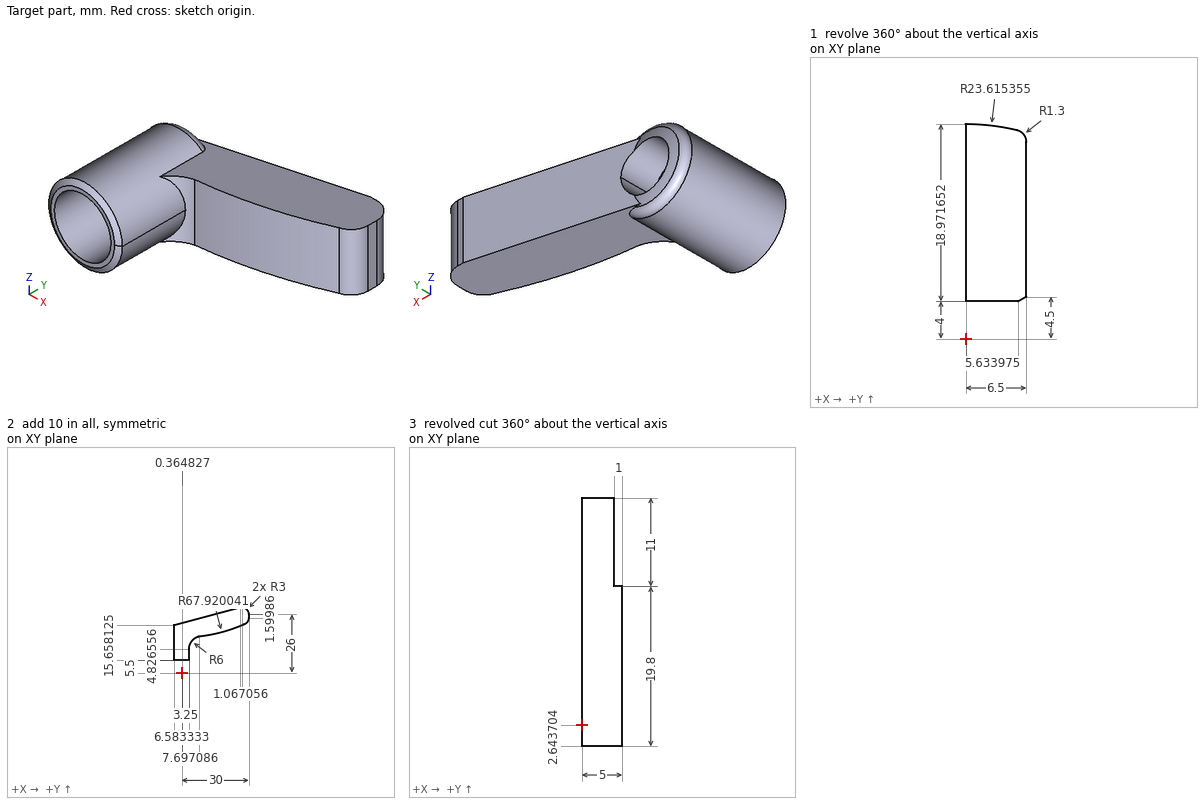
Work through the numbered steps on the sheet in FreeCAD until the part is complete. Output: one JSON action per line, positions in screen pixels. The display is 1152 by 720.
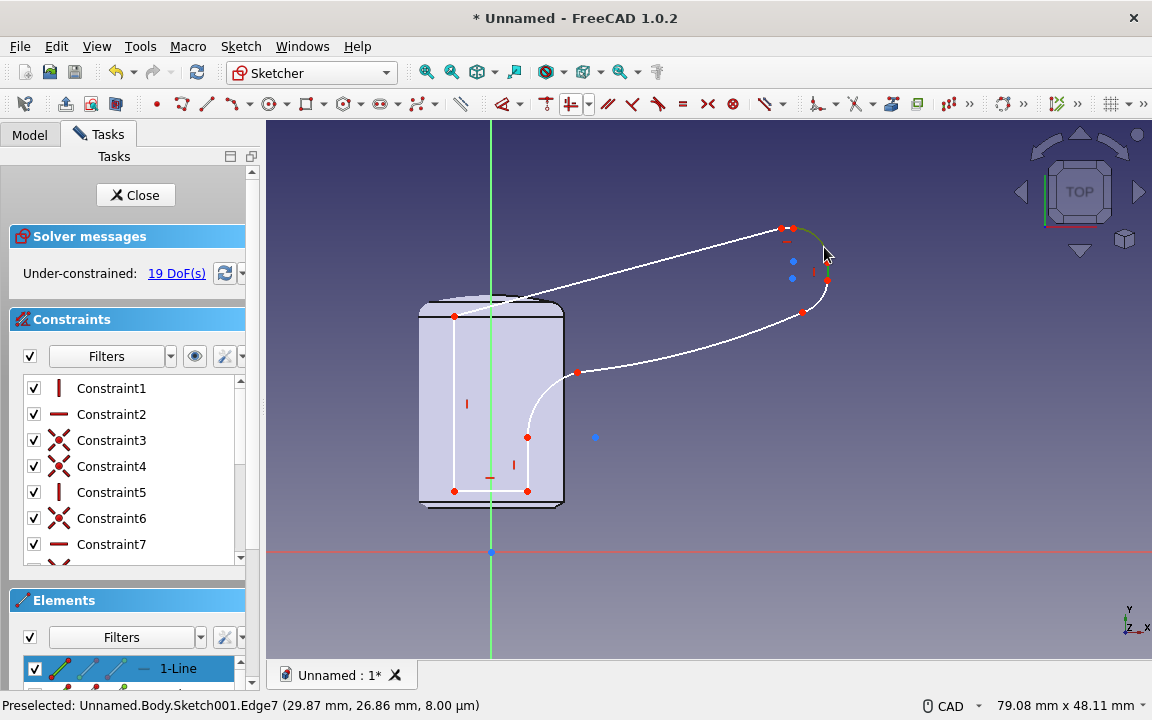
{"action": "key", "text": "t"}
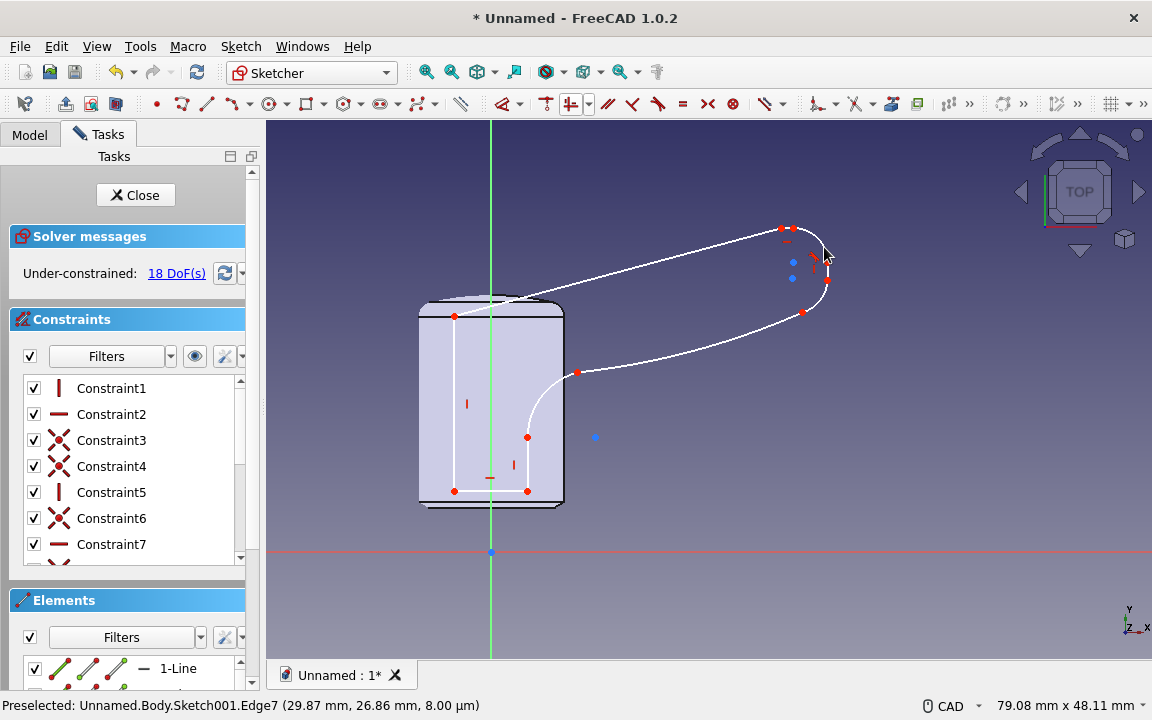
{"action": "scroll", "coordinate": [828, 271], "scroll_direction": "up", "scroll_amount": 3}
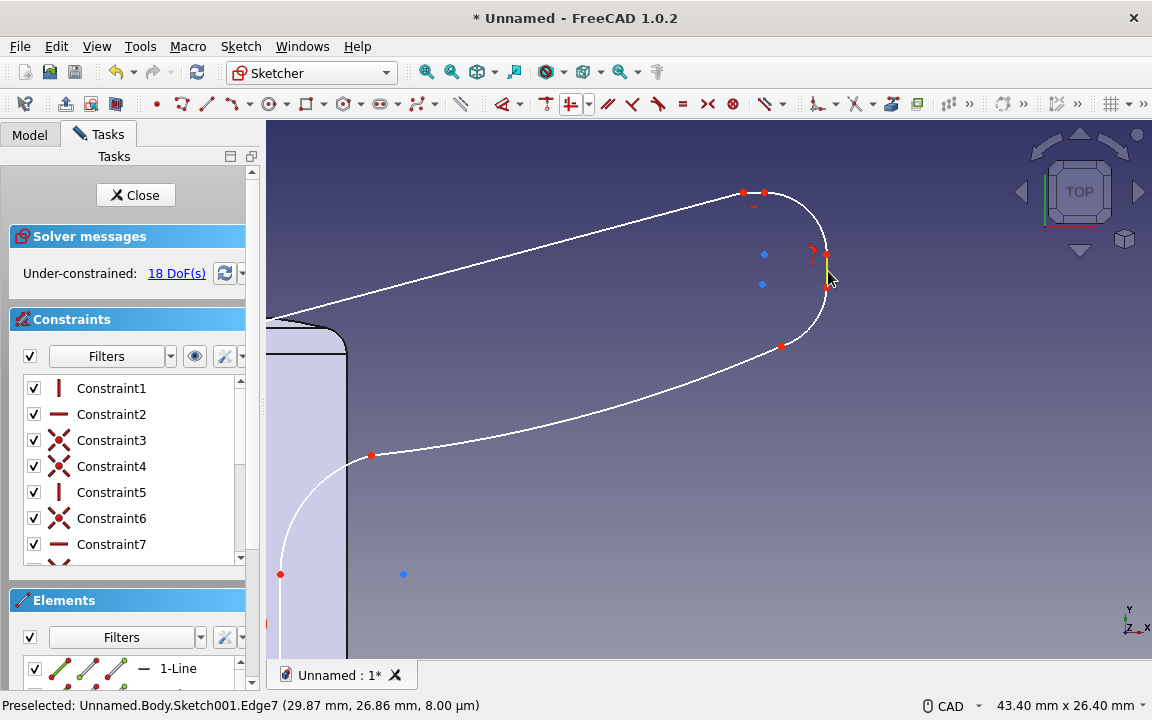
{"action": "left_click", "coordinate": [827, 271]}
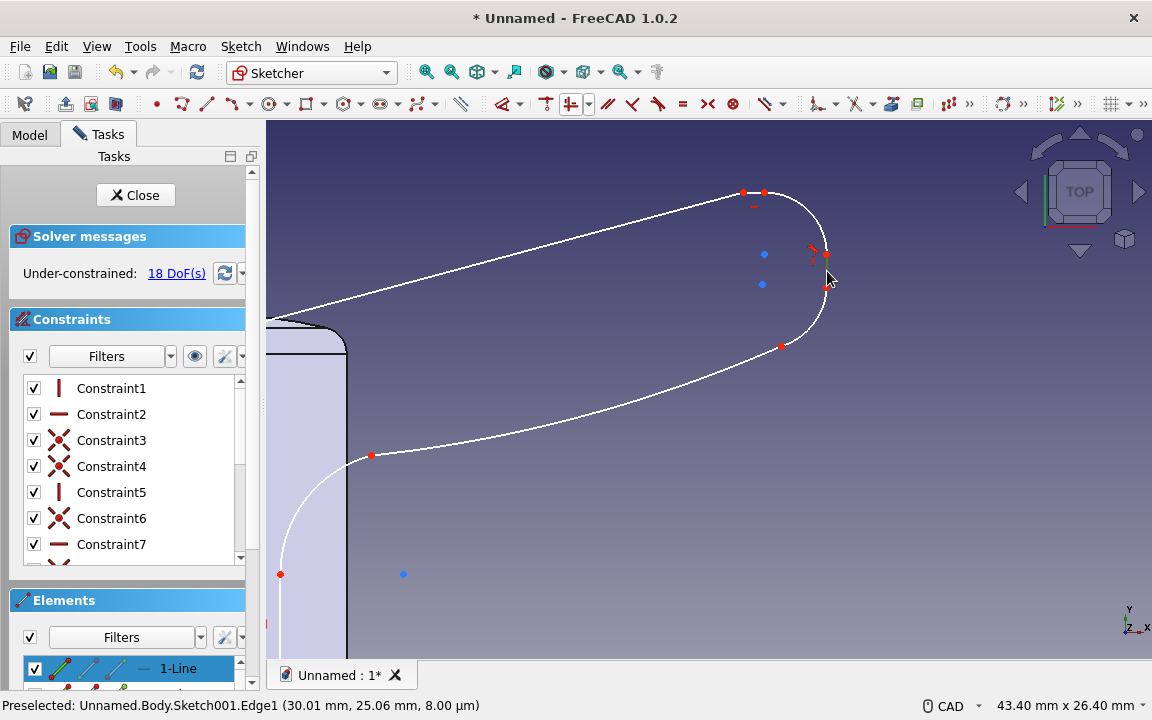
{"action": "left_click", "coordinate": [802, 335]}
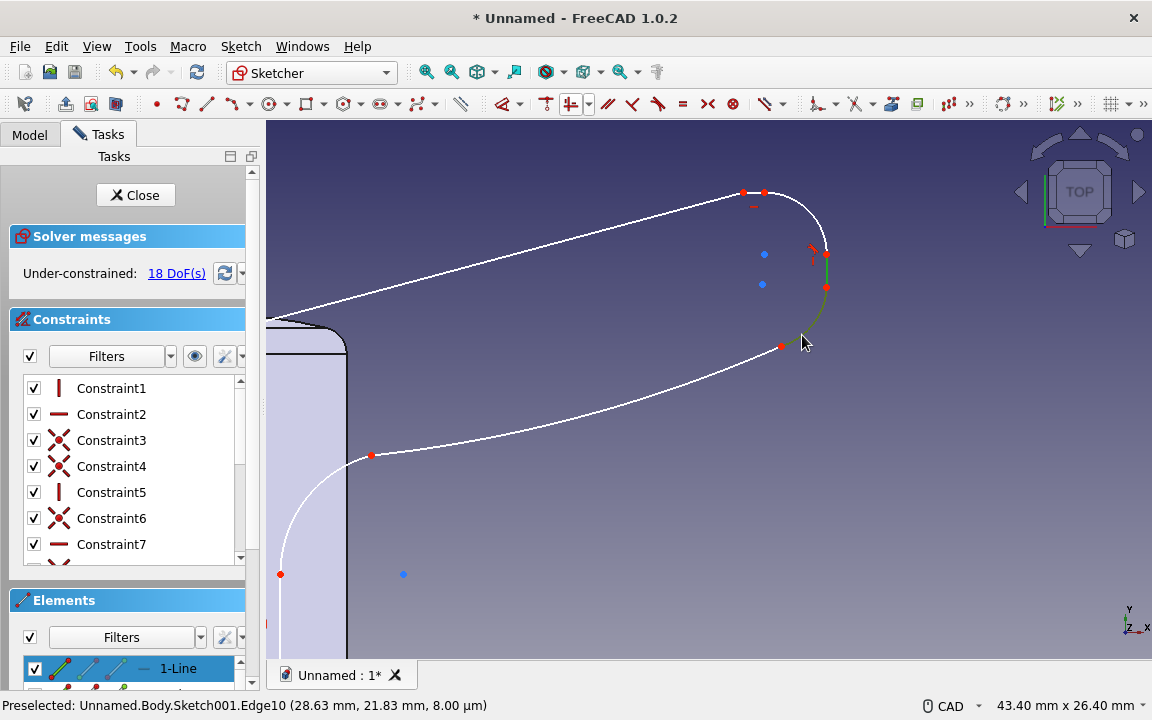
{"action": "left_click", "coordinate": [658, 104]}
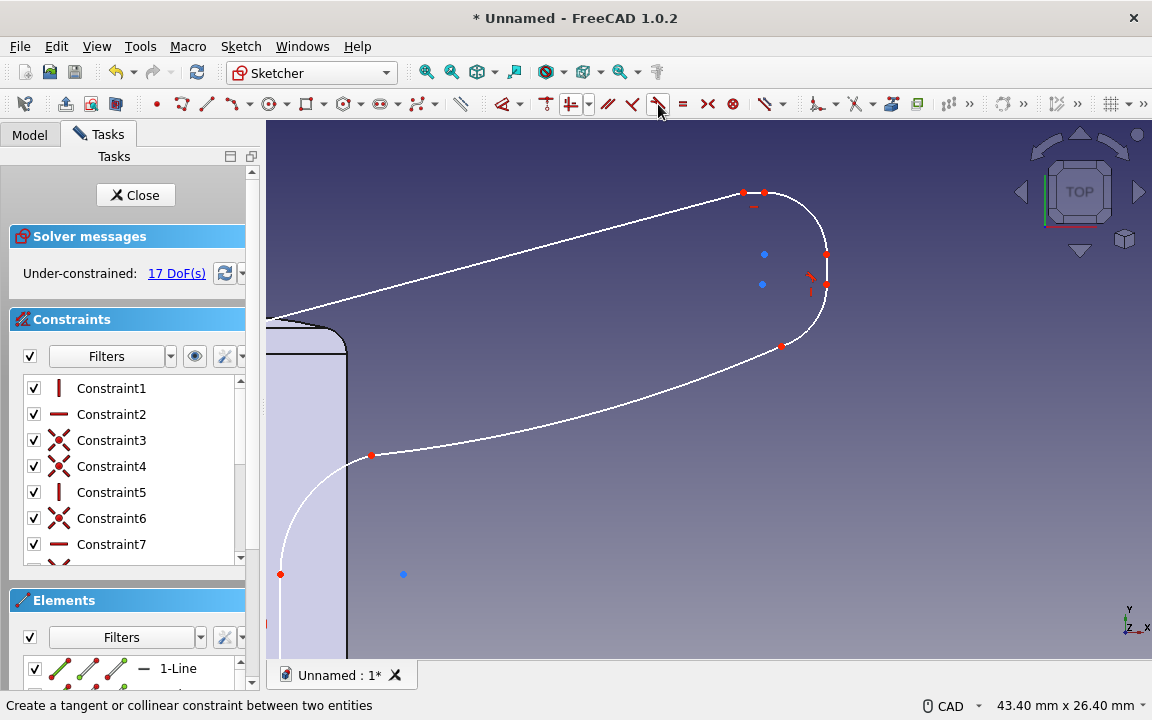
{"action": "scroll", "coordinate": [754, 193], "scroll_direction": "up", "scroll_amount": 2}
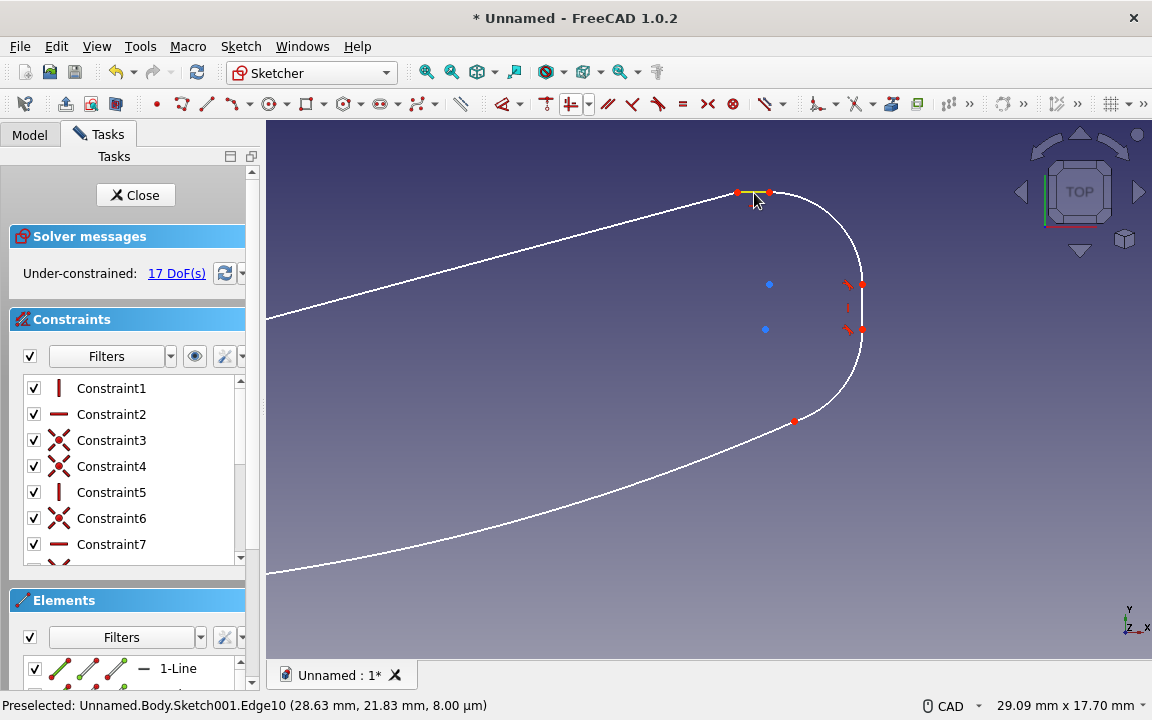
{"action": "left_click", "coordinate": [754, 192]}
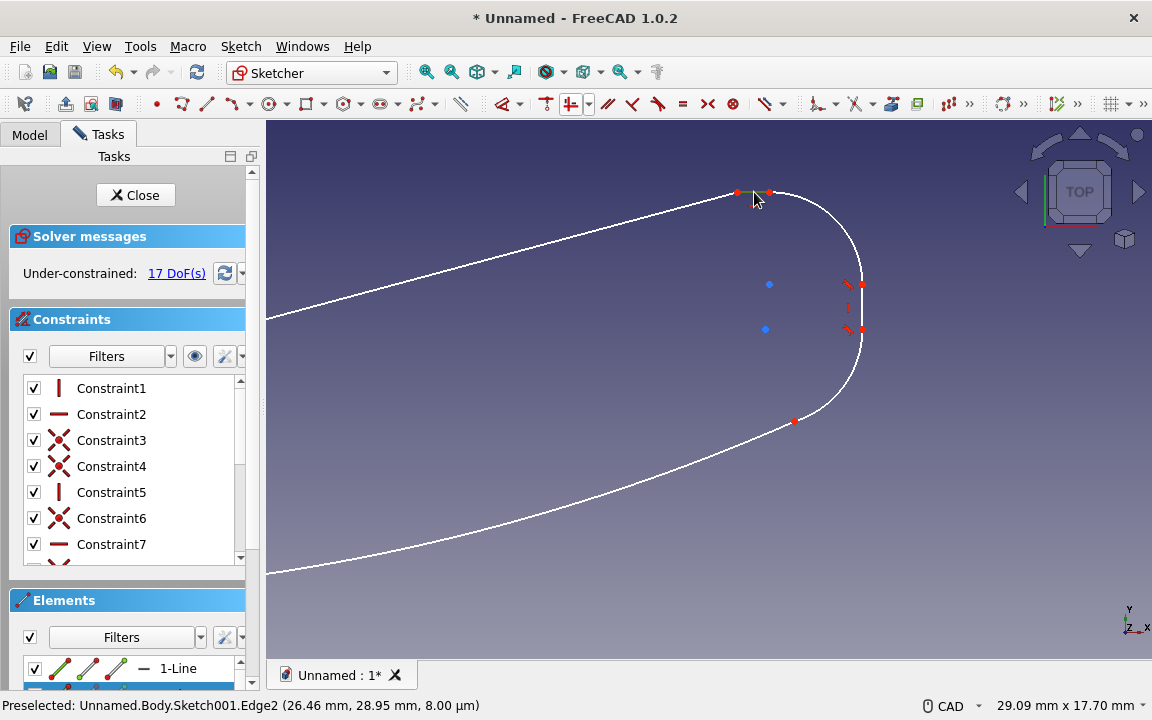
{"action": "left_click", "coordinate": [852, 243]}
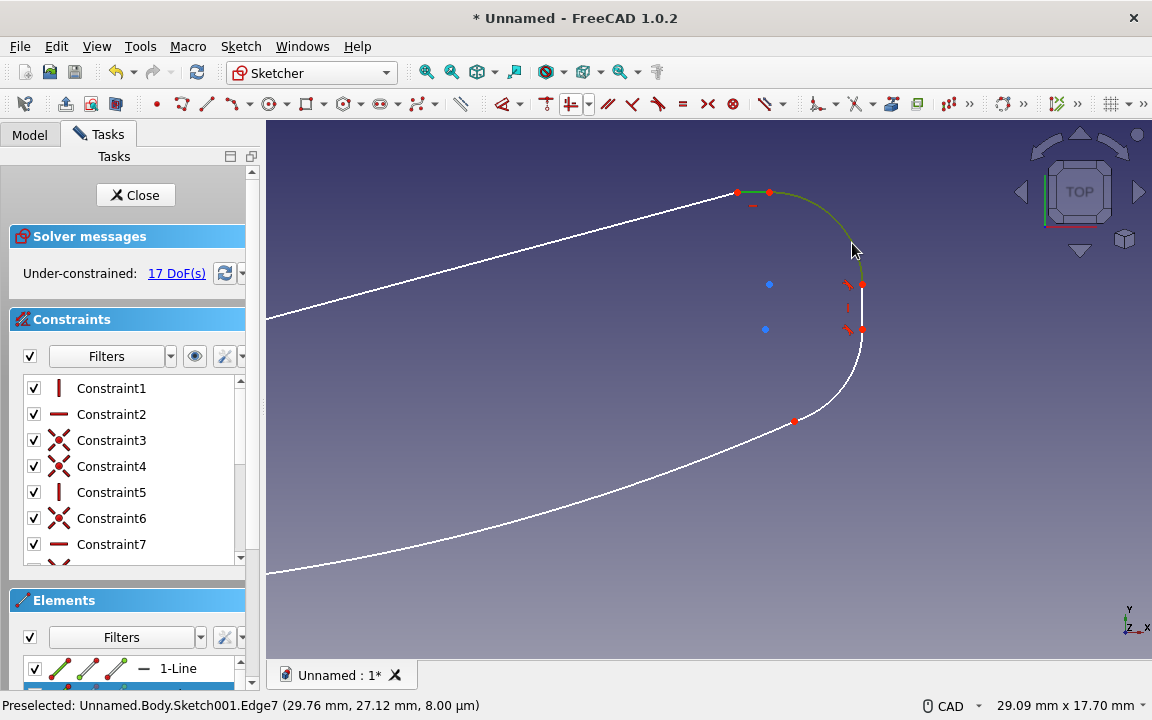
{"action": "key", "text": "t"}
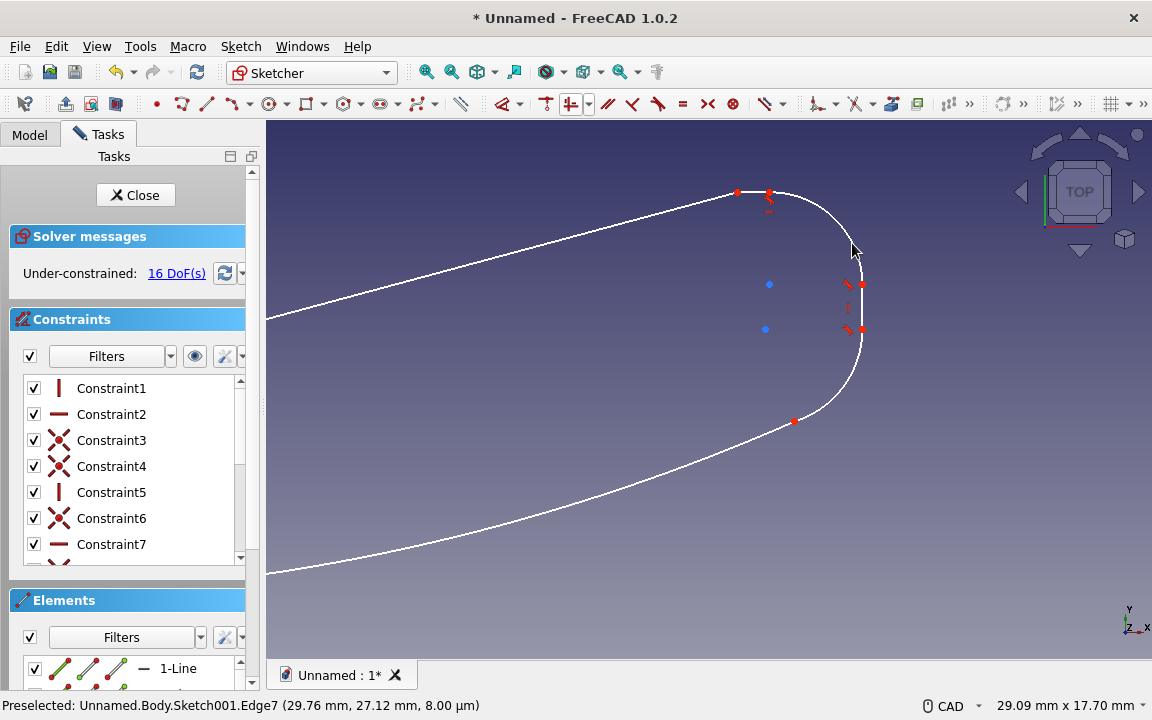
{"action": "scroll", "coordinate": [807, 248], "scroll_direction": "down", "scroll_amount": 5}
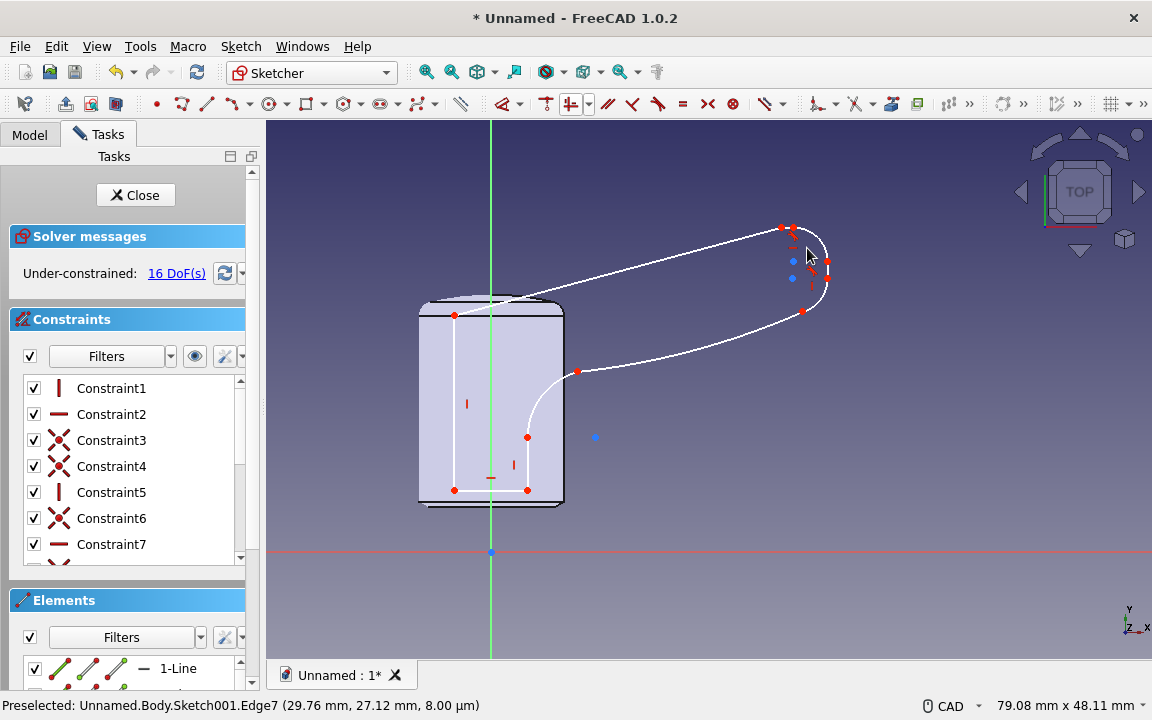
{"action": "left_click", "coordinate": [528, 475]}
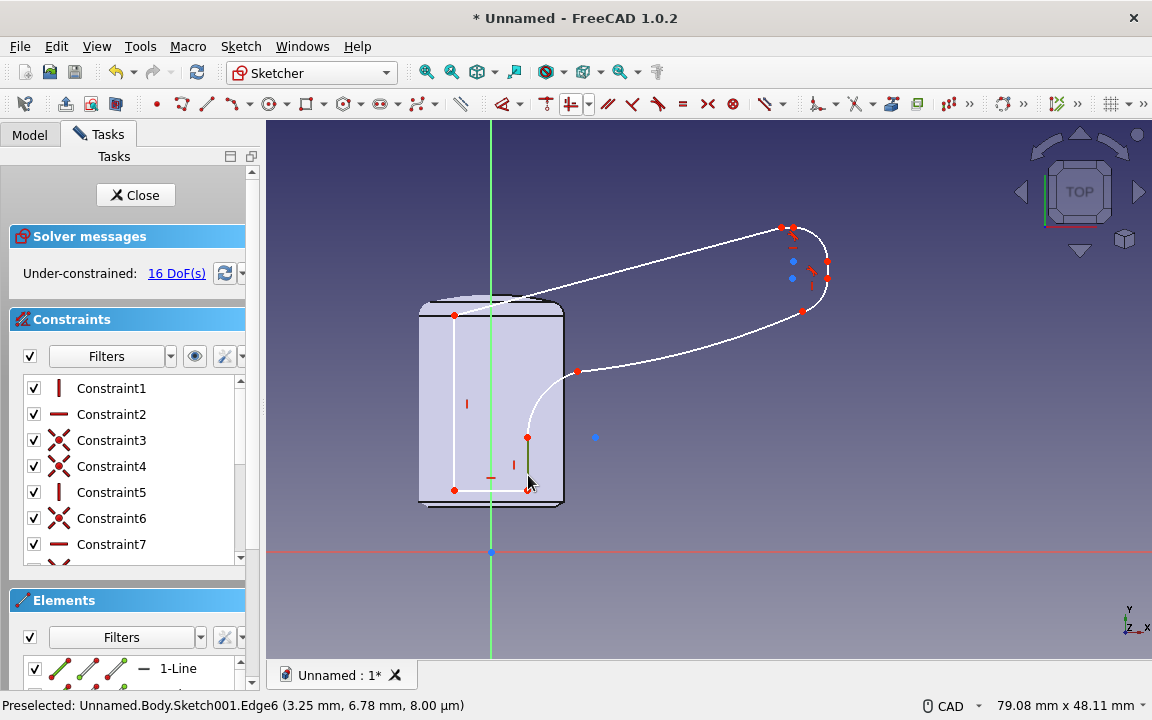
{"action": "left_click", "coordinate": [554, 384]}